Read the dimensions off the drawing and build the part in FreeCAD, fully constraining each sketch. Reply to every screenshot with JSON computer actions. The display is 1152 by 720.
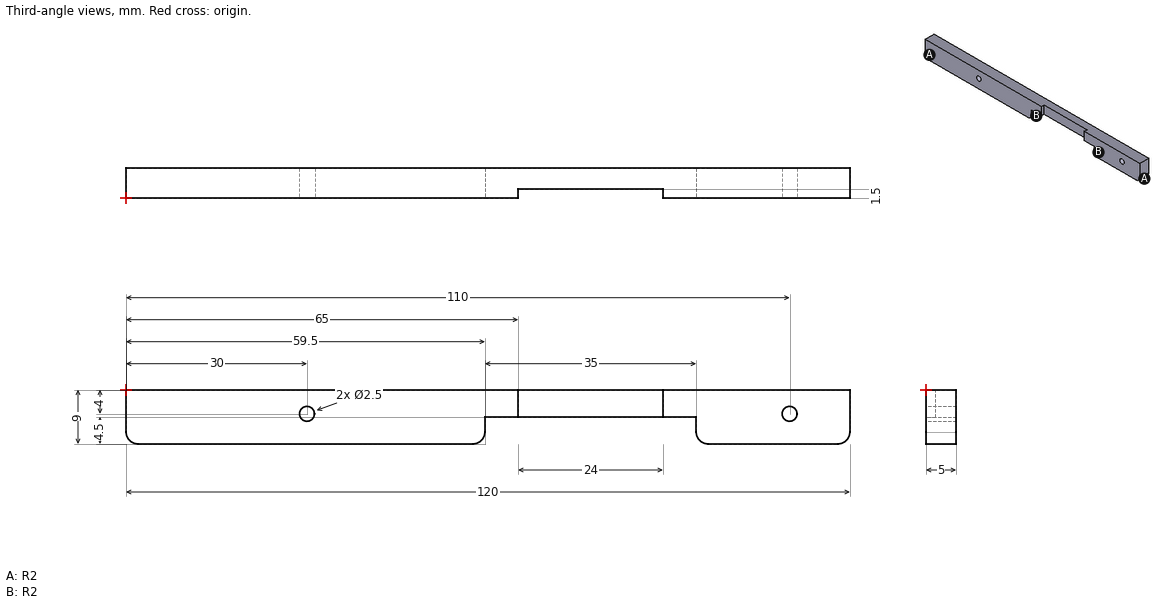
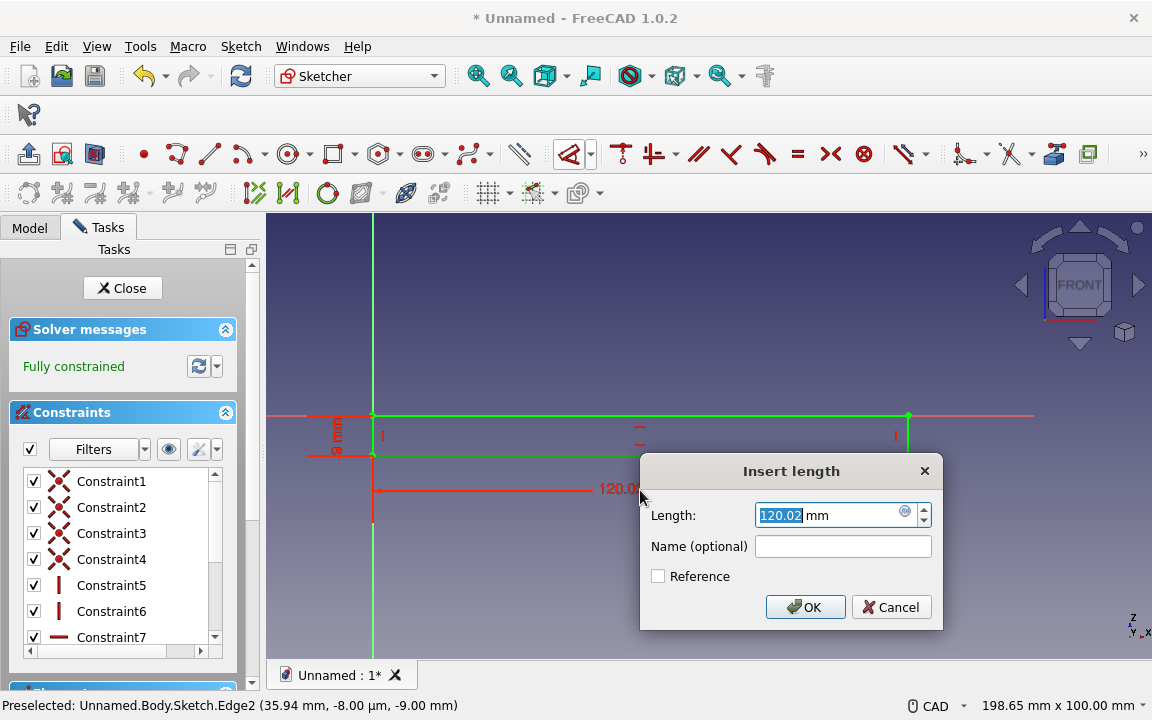
{"action": "type", "text": "120"}
{"action": "key", "text": "Return"}
{"action": "key", "text": "Escape"}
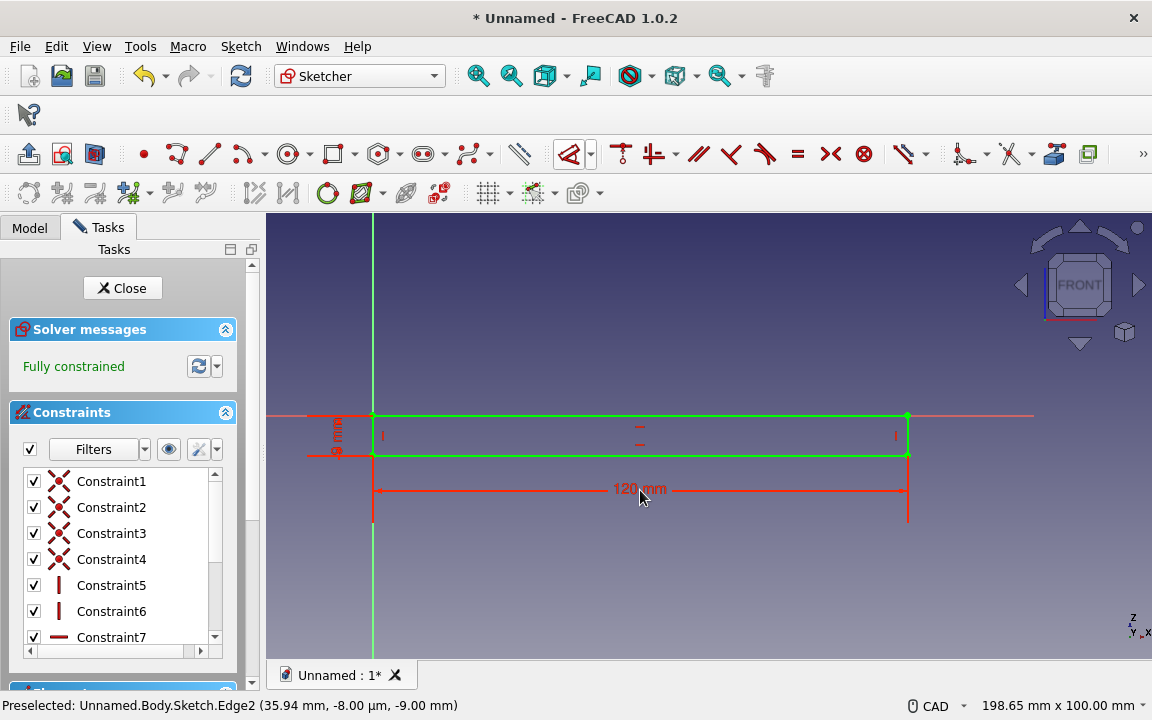
{"action": "left_click", "coordinate": [123, 288]}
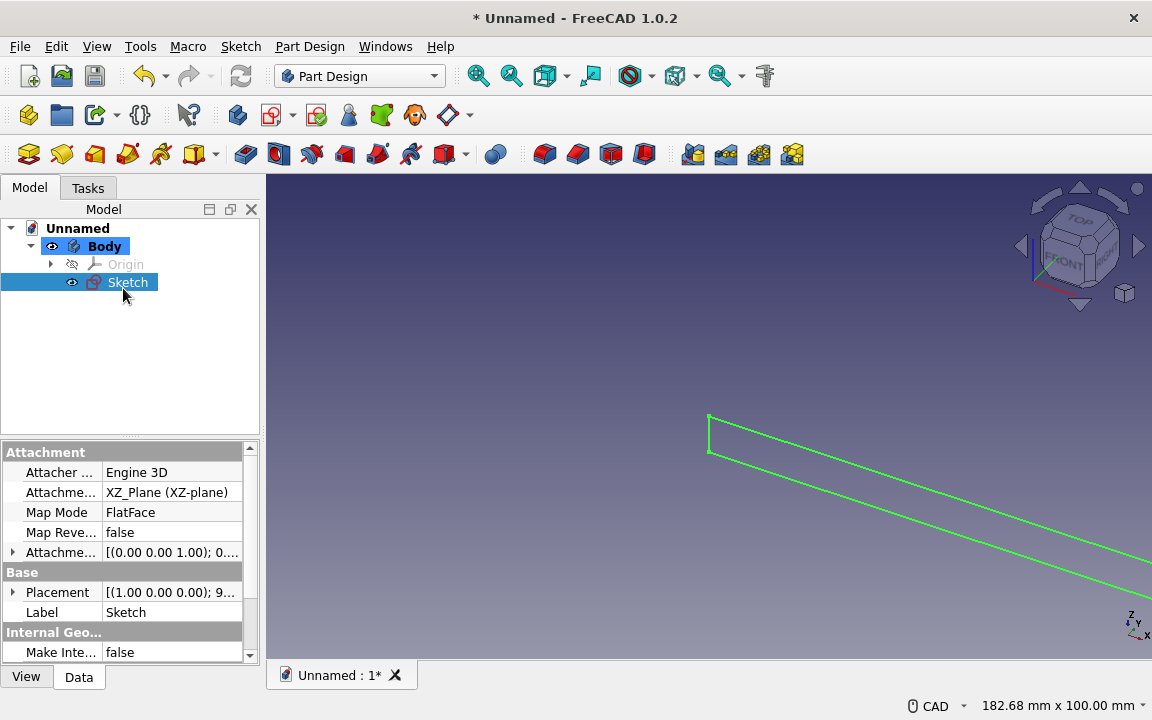
{"action": "left_click", "coordinate": [29, 154]}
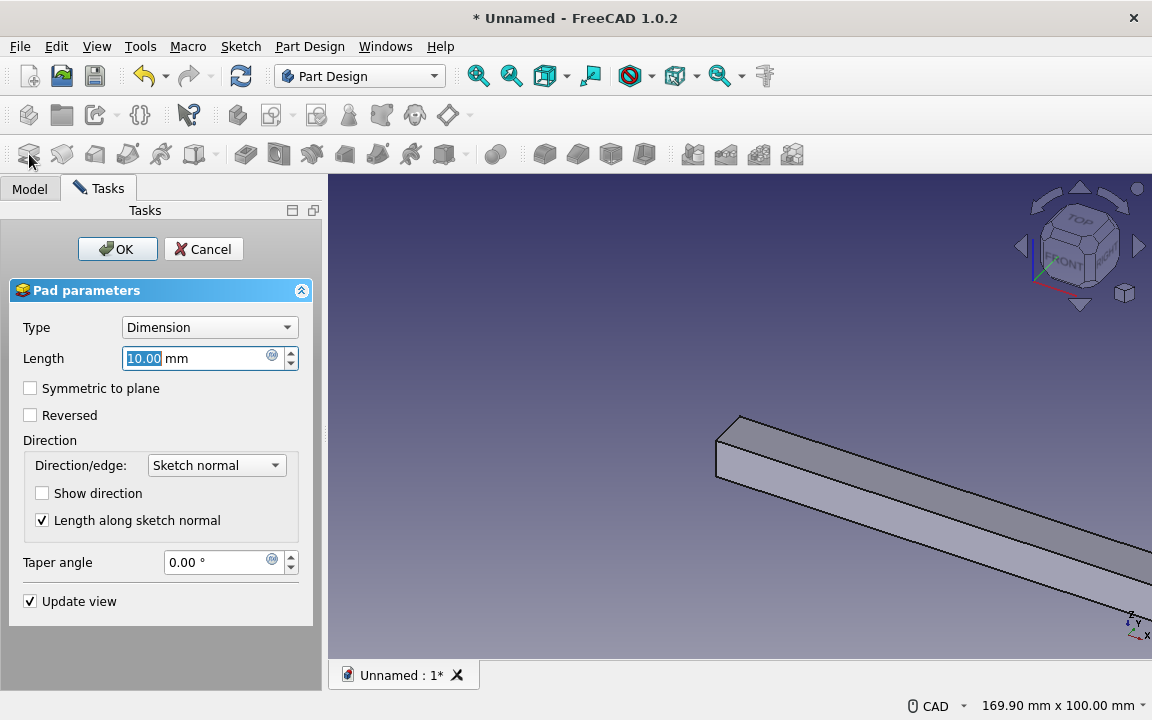
{"action": "type", "text": "5"}
{"action": "key", "text": "Tab"}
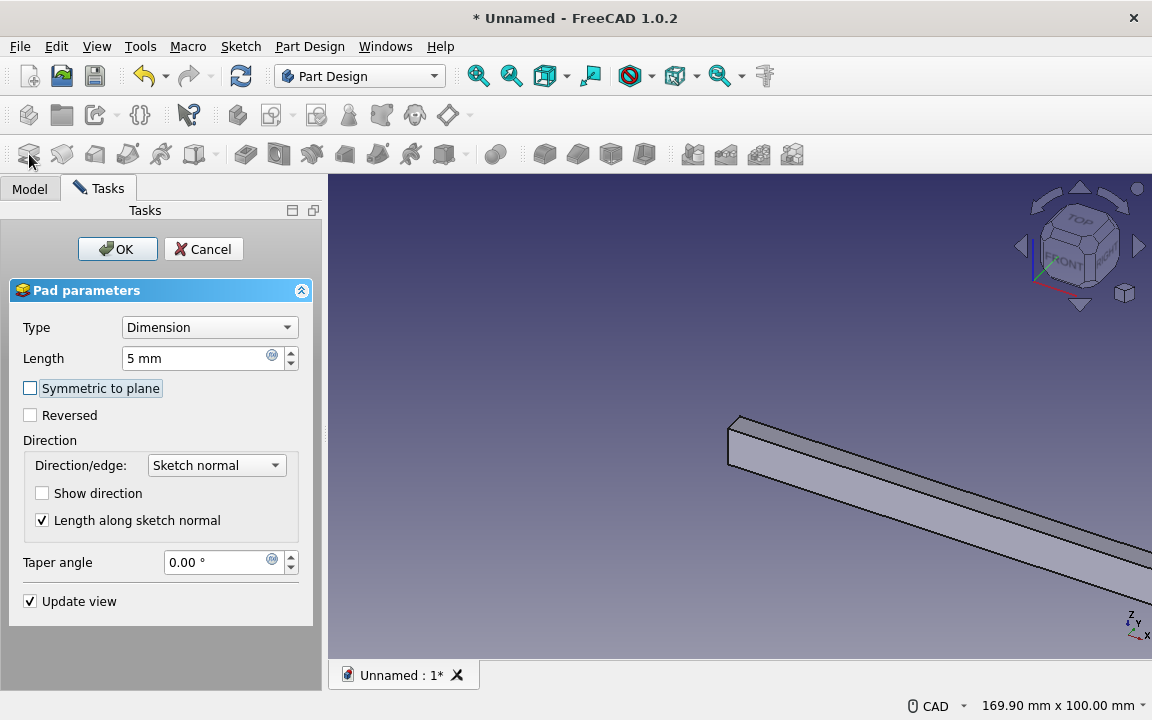
{"action": "left_click", "coordinate": [31, 415]}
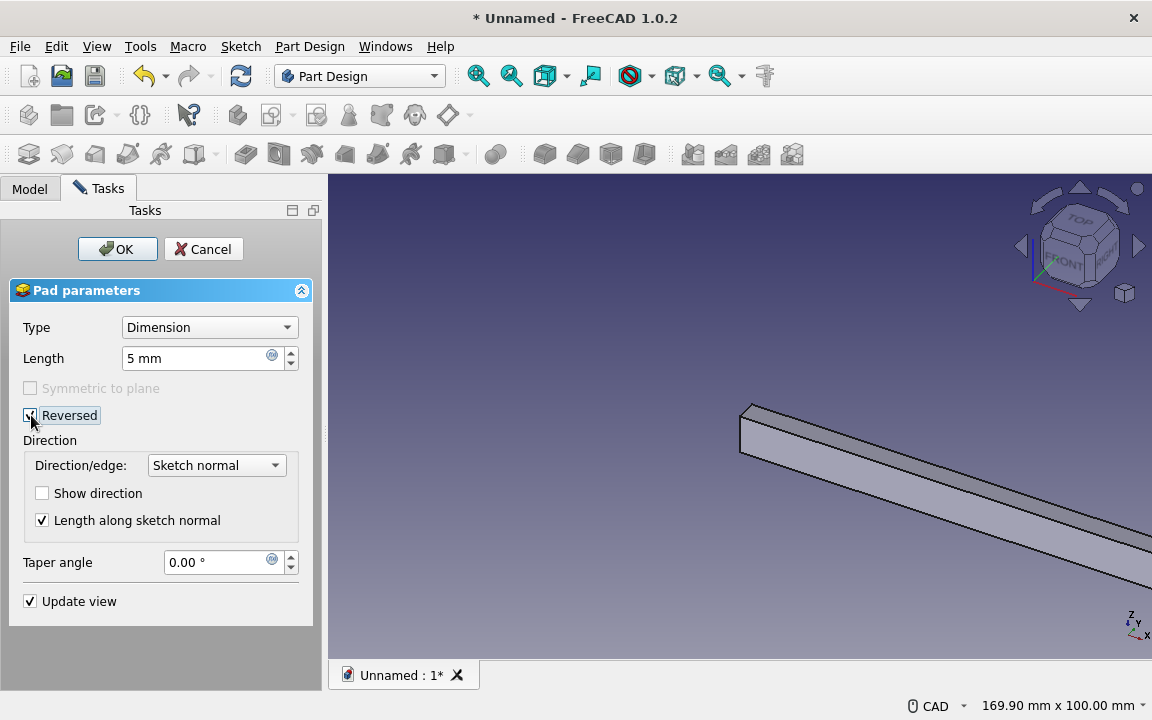
{"action": "left_click", "coordinate": [118, 249]}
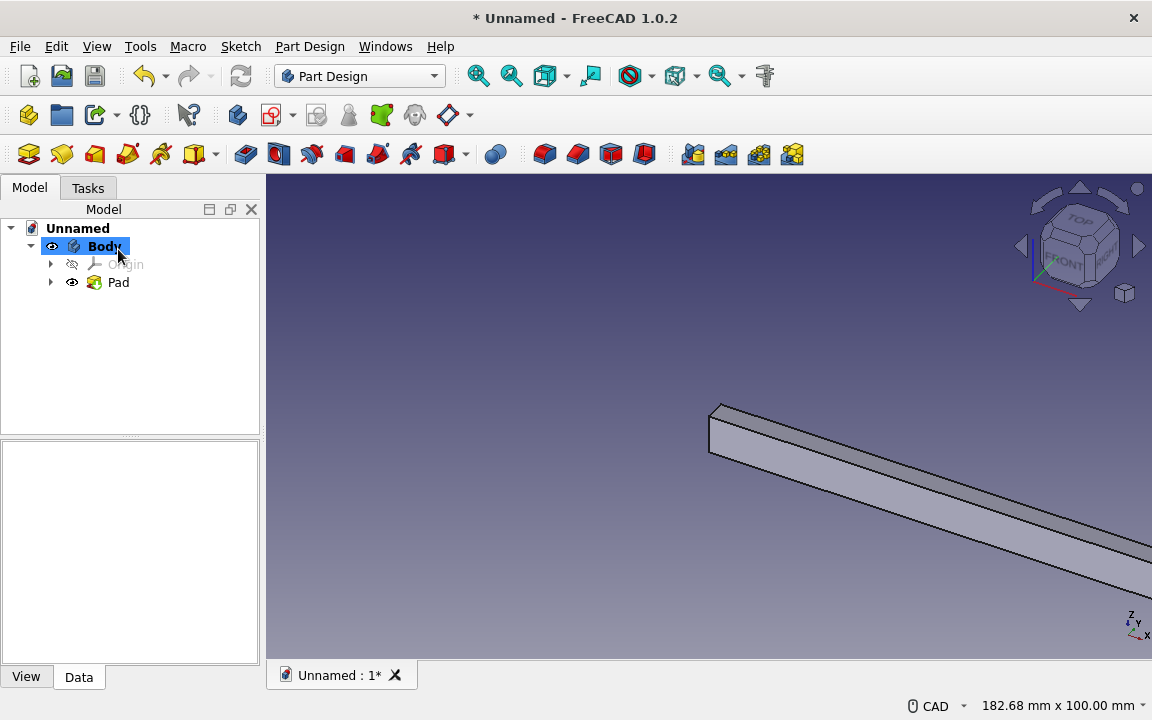
{"action": "key", "text": "v f"}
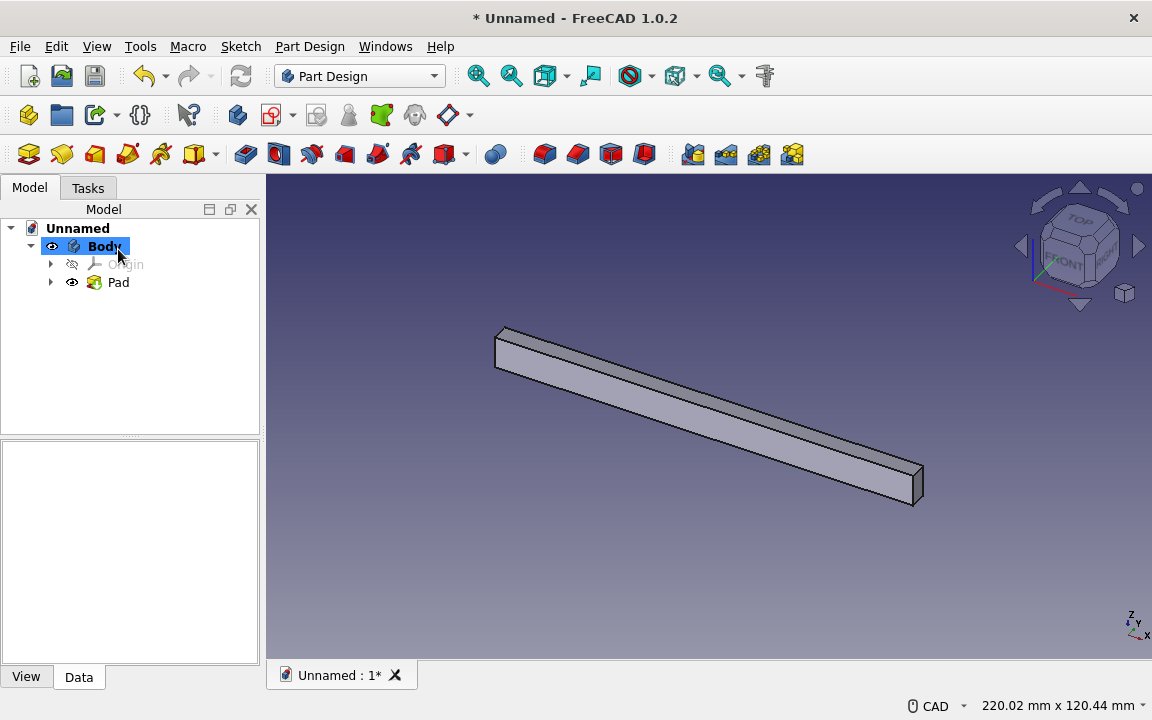
{"action": "key", "text": "4"}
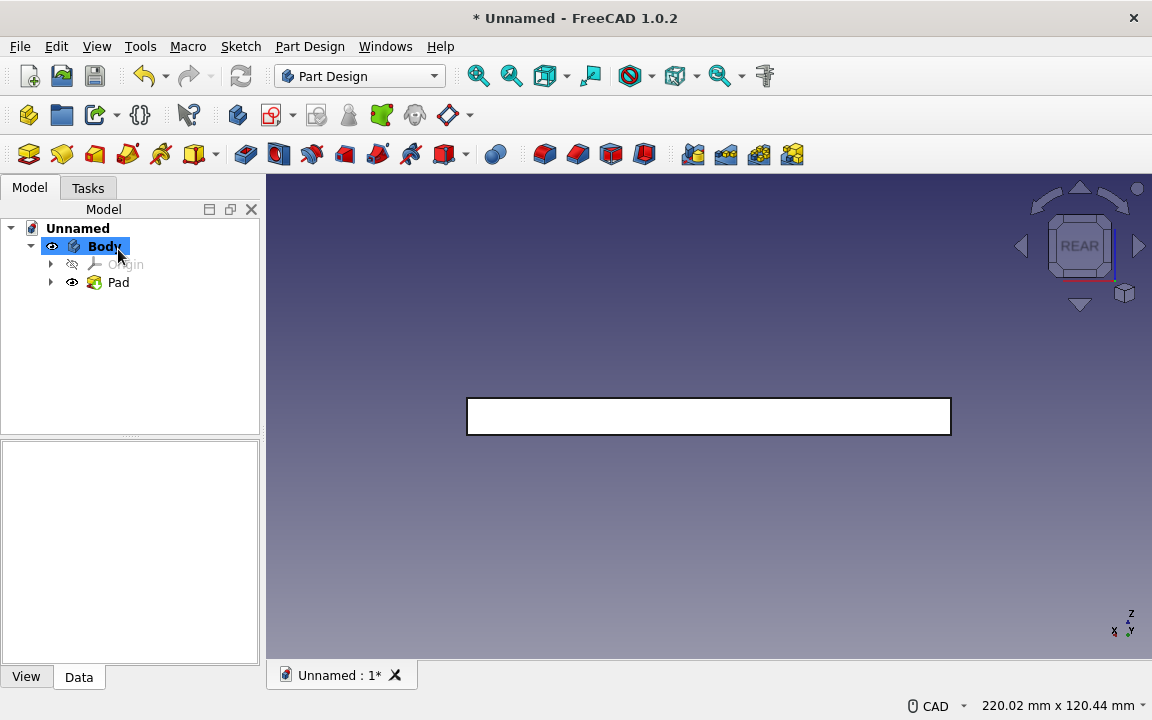
{"action": "left_click", "coordinate": [502, 416]}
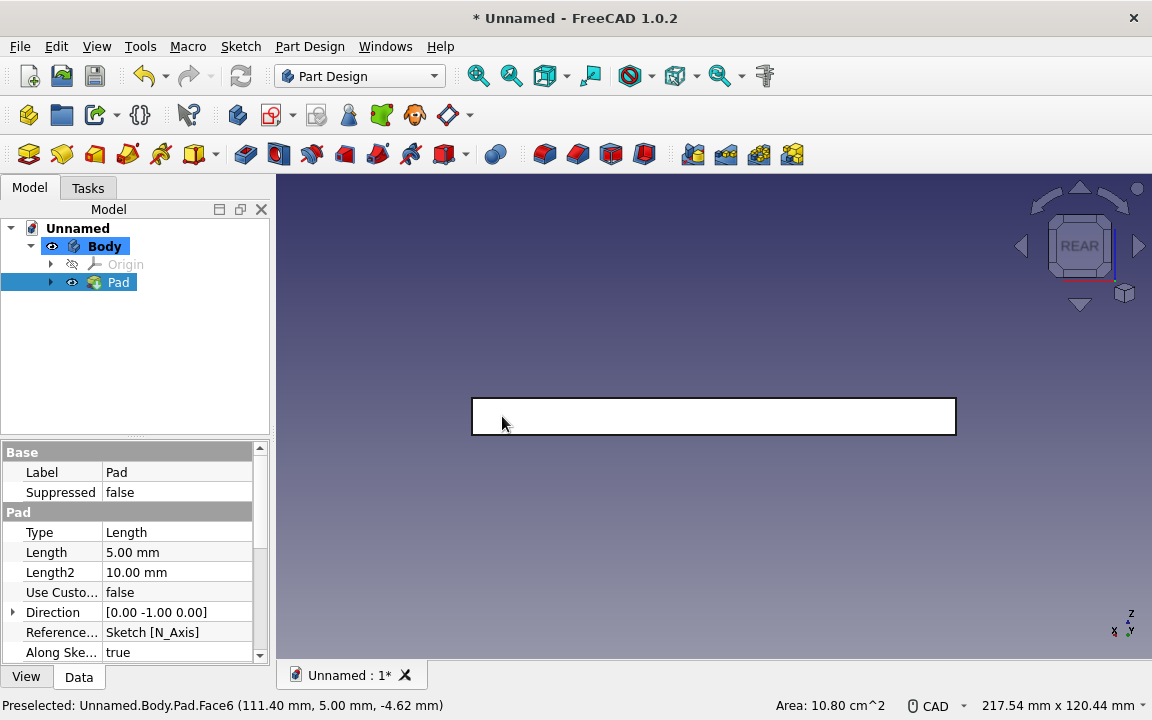
{"action": "left_click", "coordinate": [270, 116]}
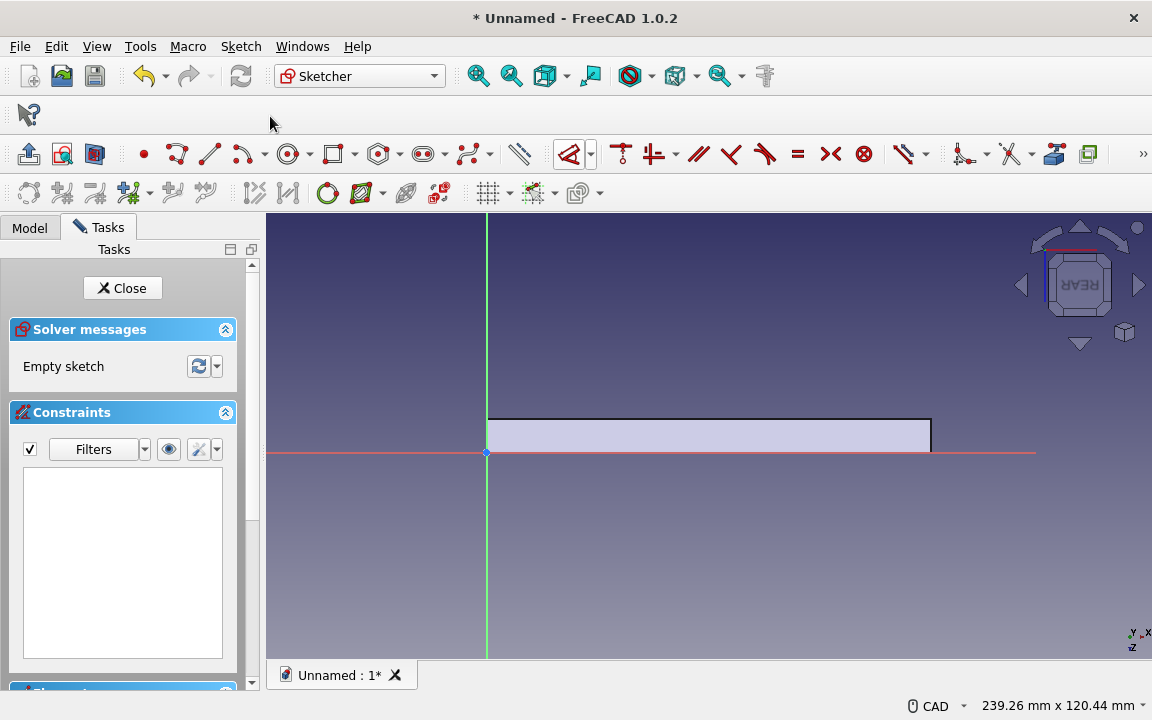
{"action": "key", "text": "g c"}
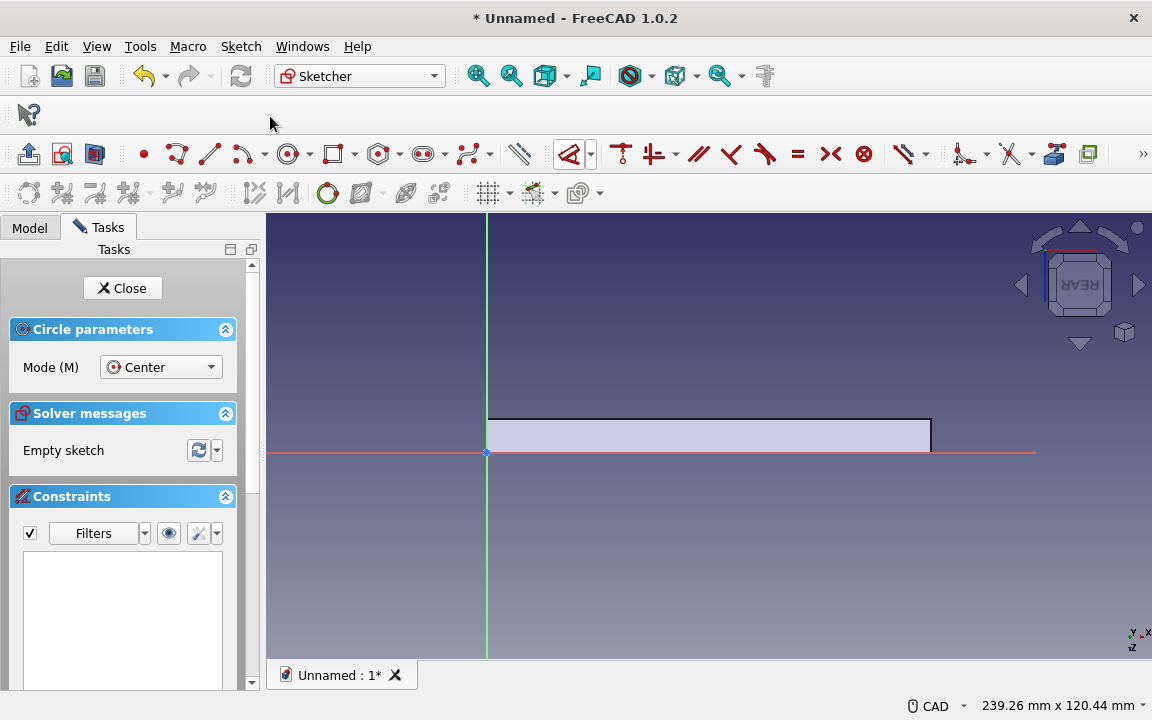
{"action": "scroll", "coordinate": [598, 438], "scroll_direction": "up", "scroll_amount": 8}